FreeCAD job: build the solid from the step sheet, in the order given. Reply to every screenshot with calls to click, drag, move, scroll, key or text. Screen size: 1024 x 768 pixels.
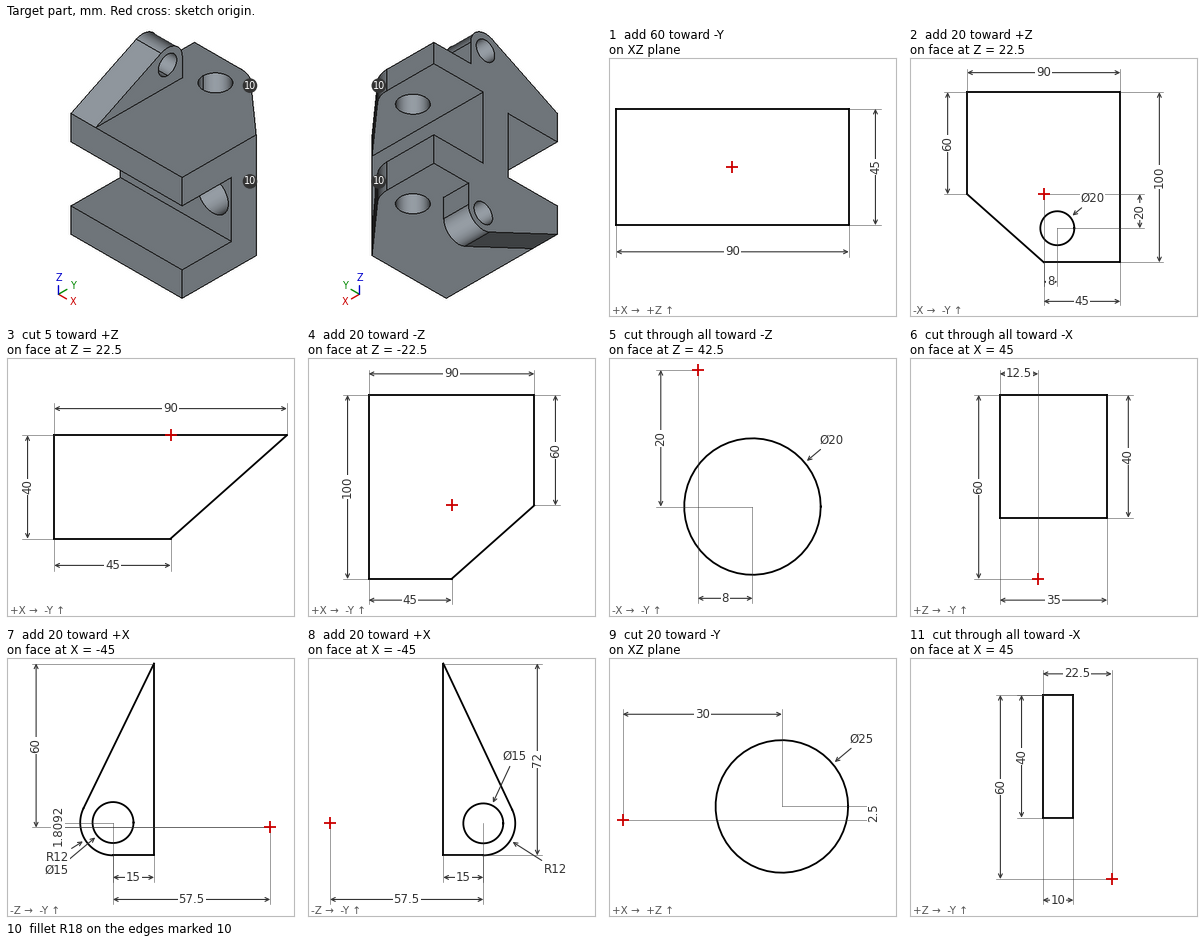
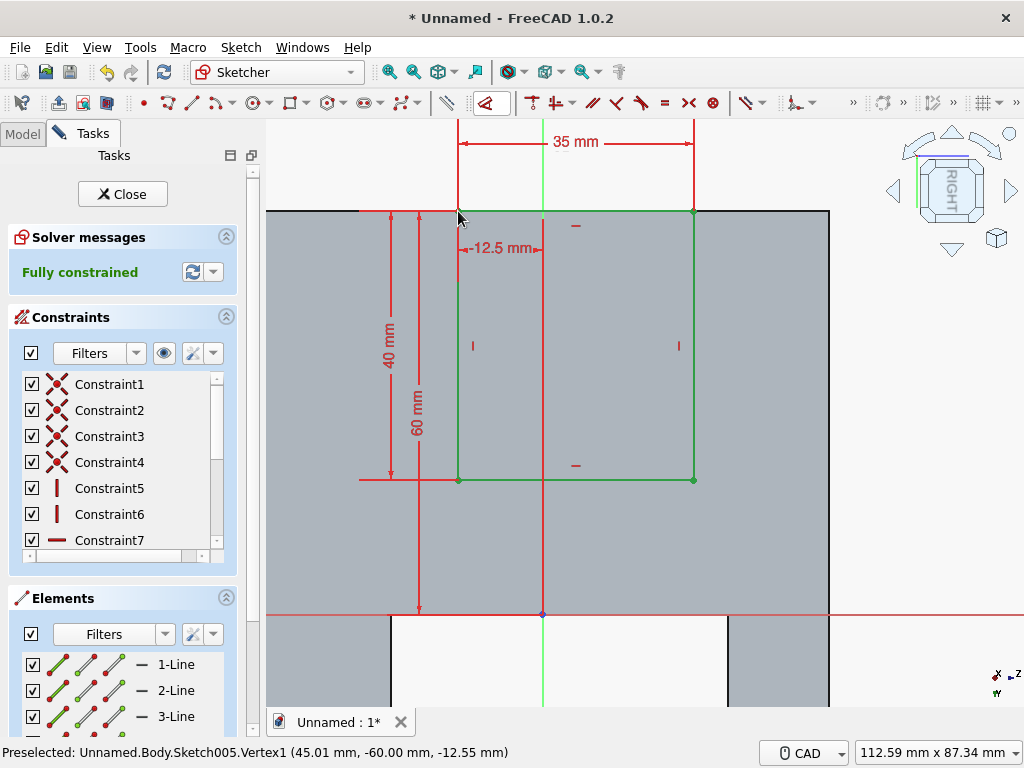
click(123, 194)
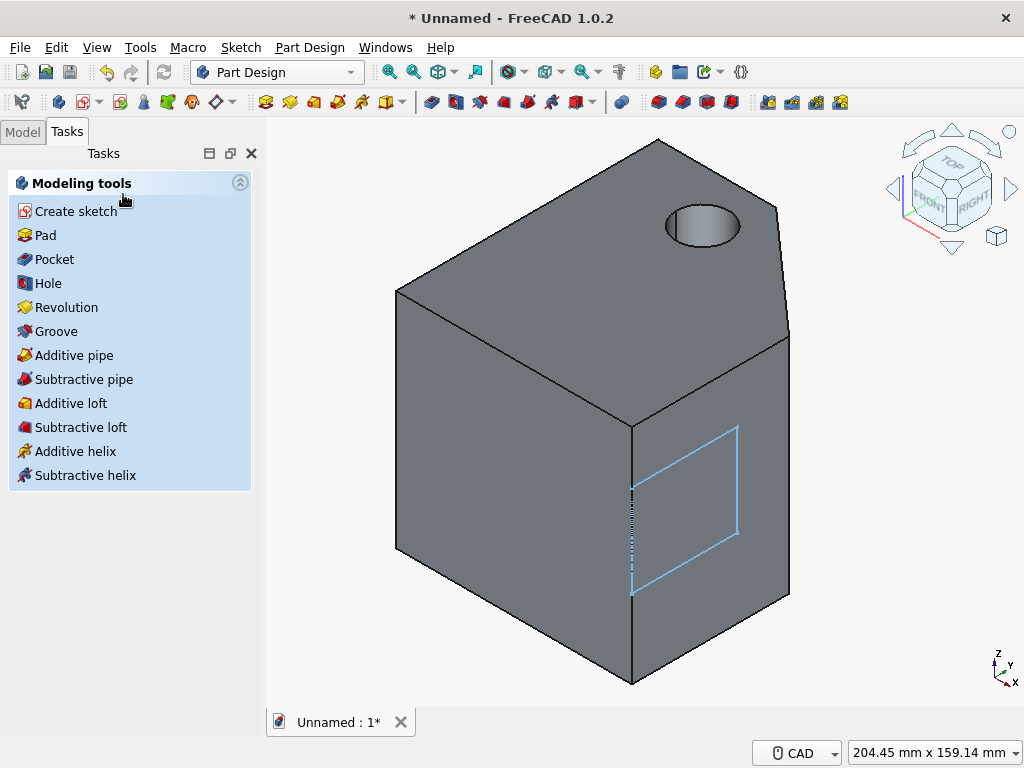
click(432, 102)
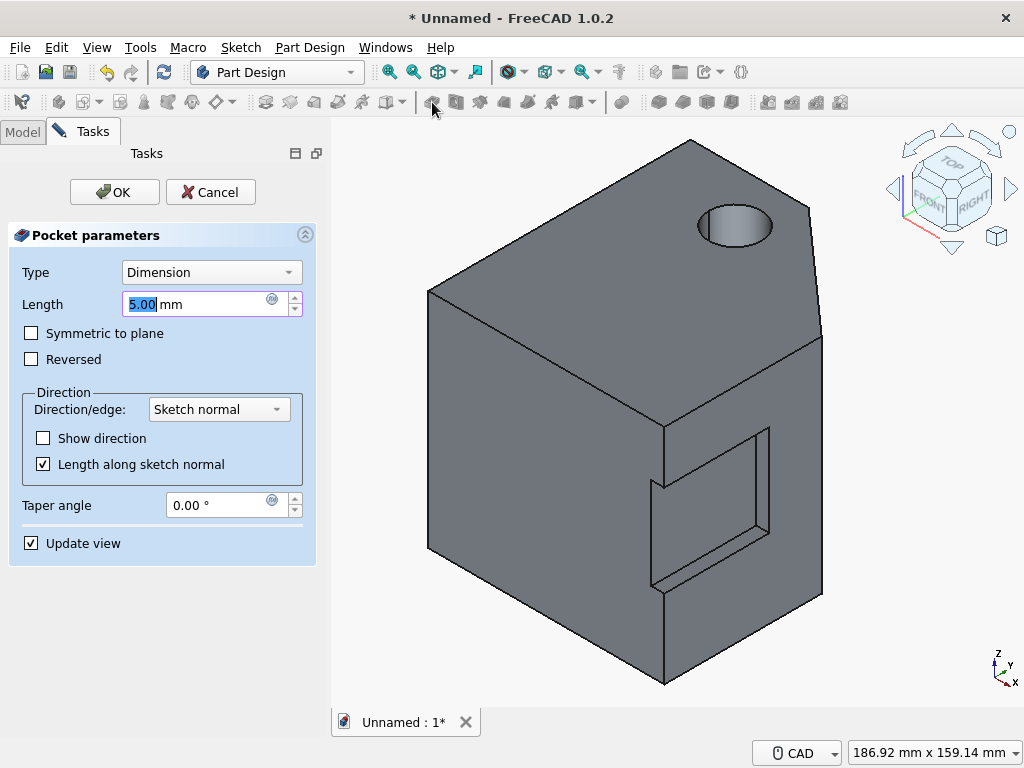
click(212, 272)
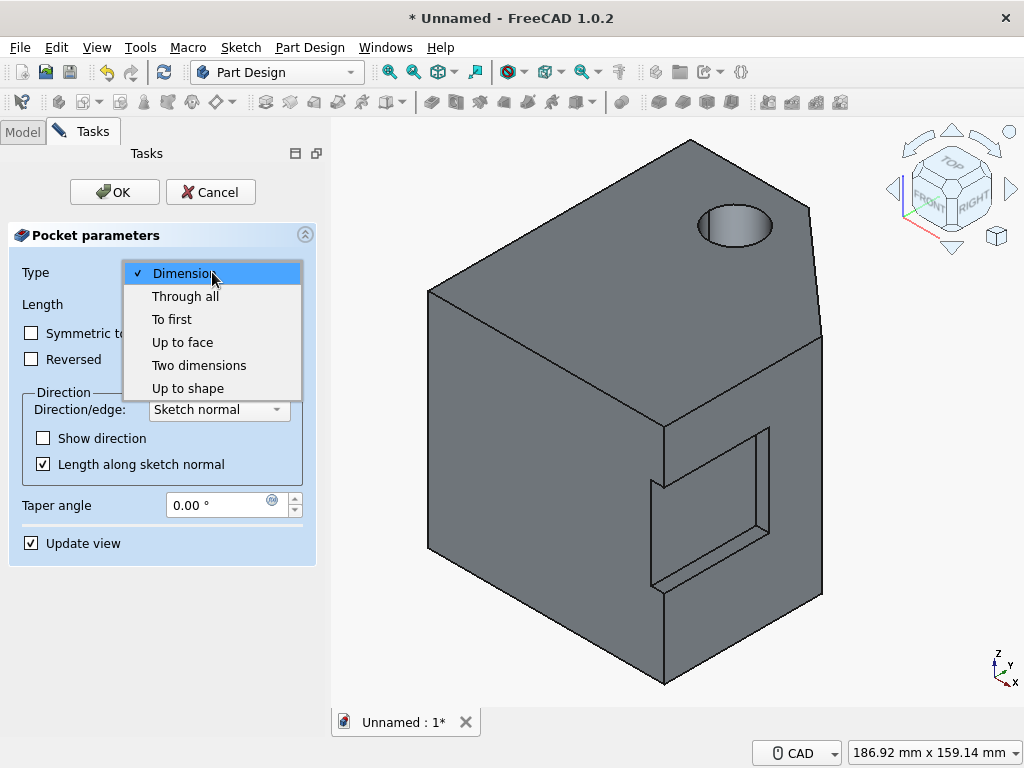
click(212, 296)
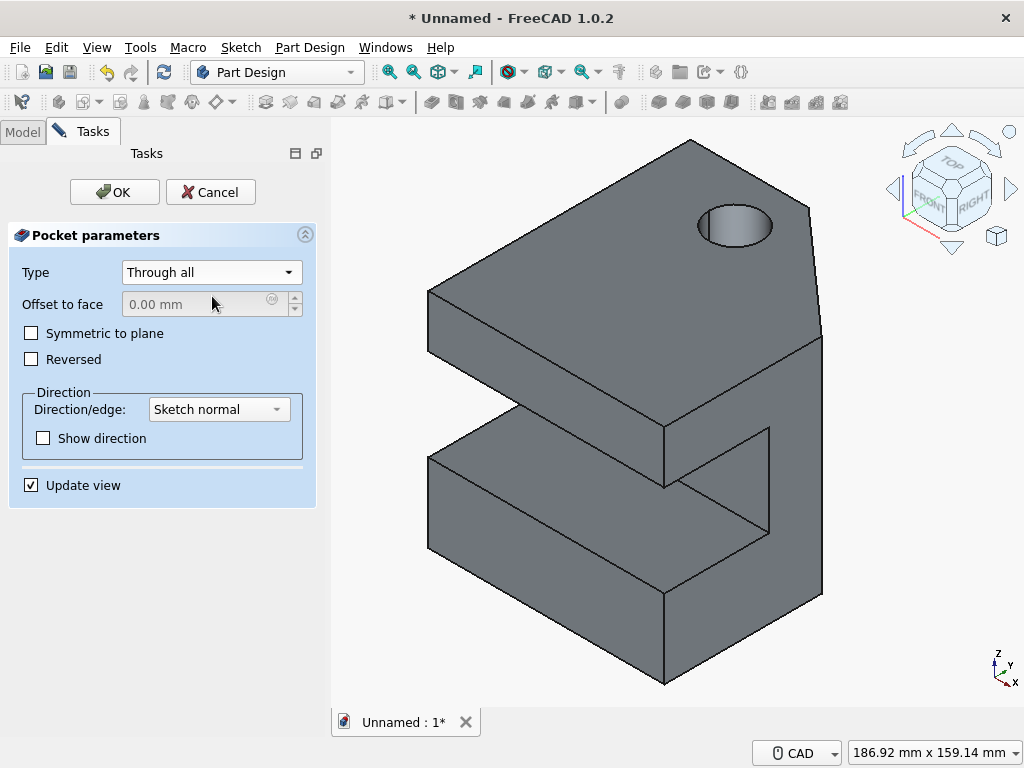
click(115, 192)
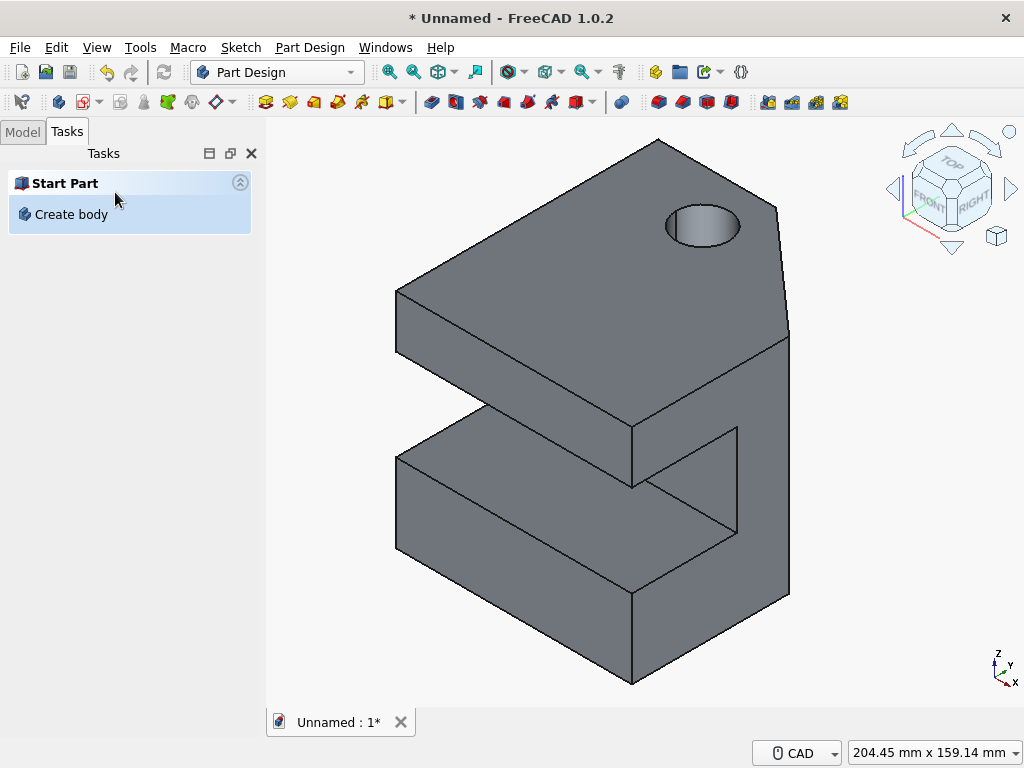
key(6)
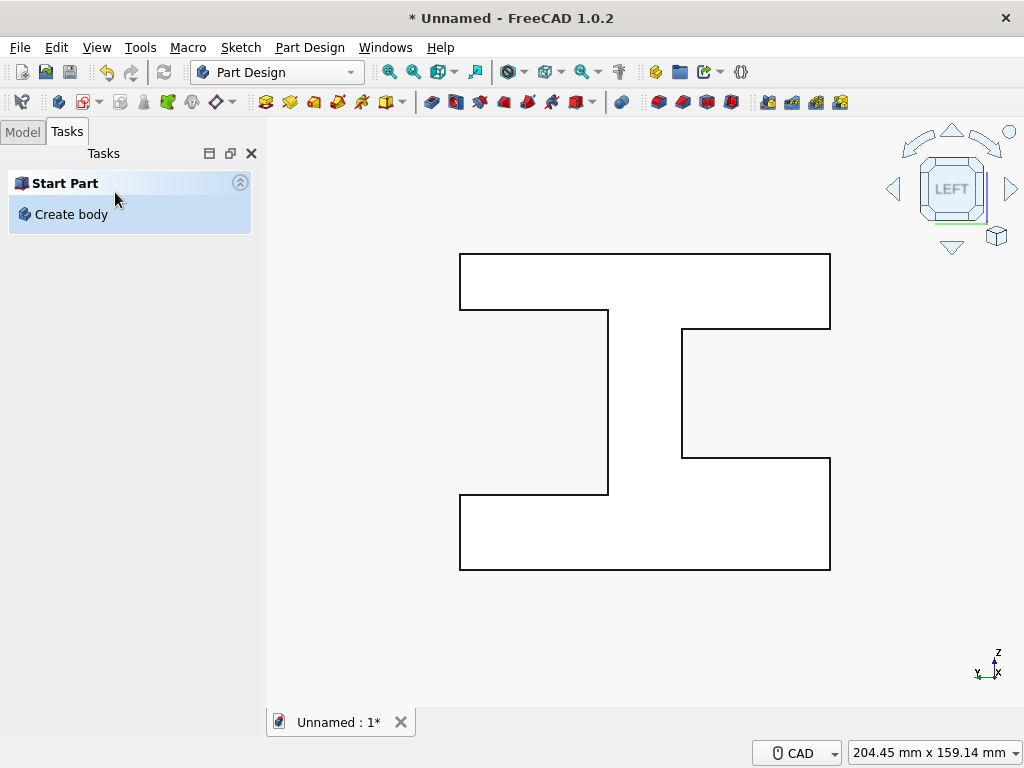
click(698, 501)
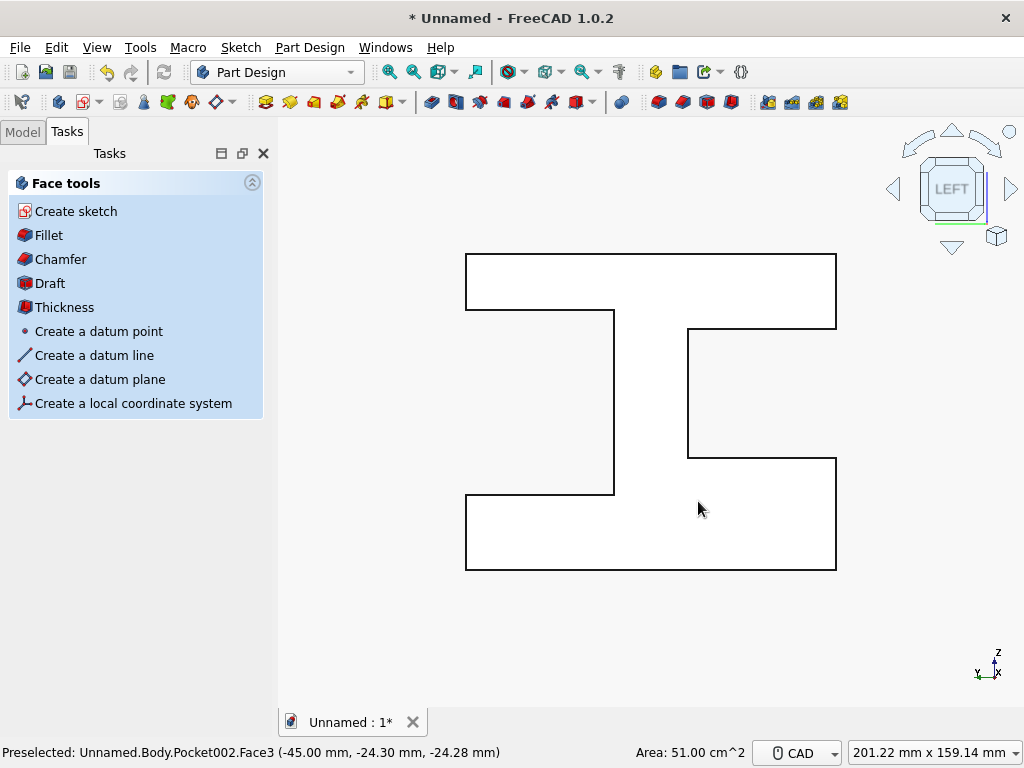
click(84, 102)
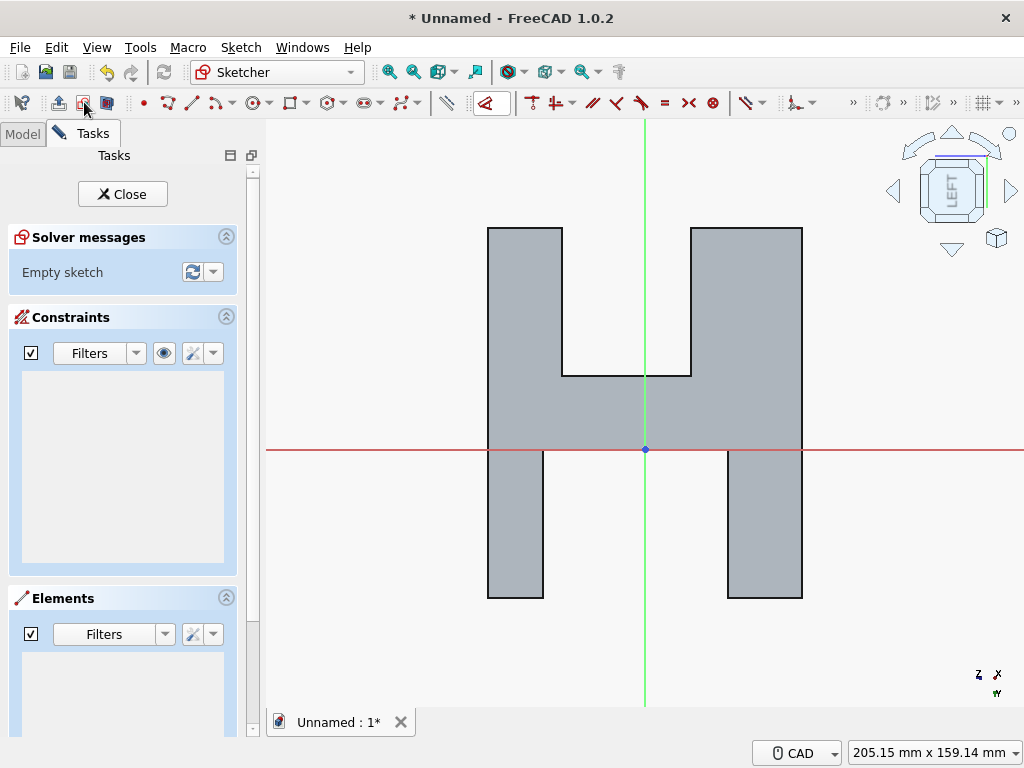
scroll(402, 246, up, 2)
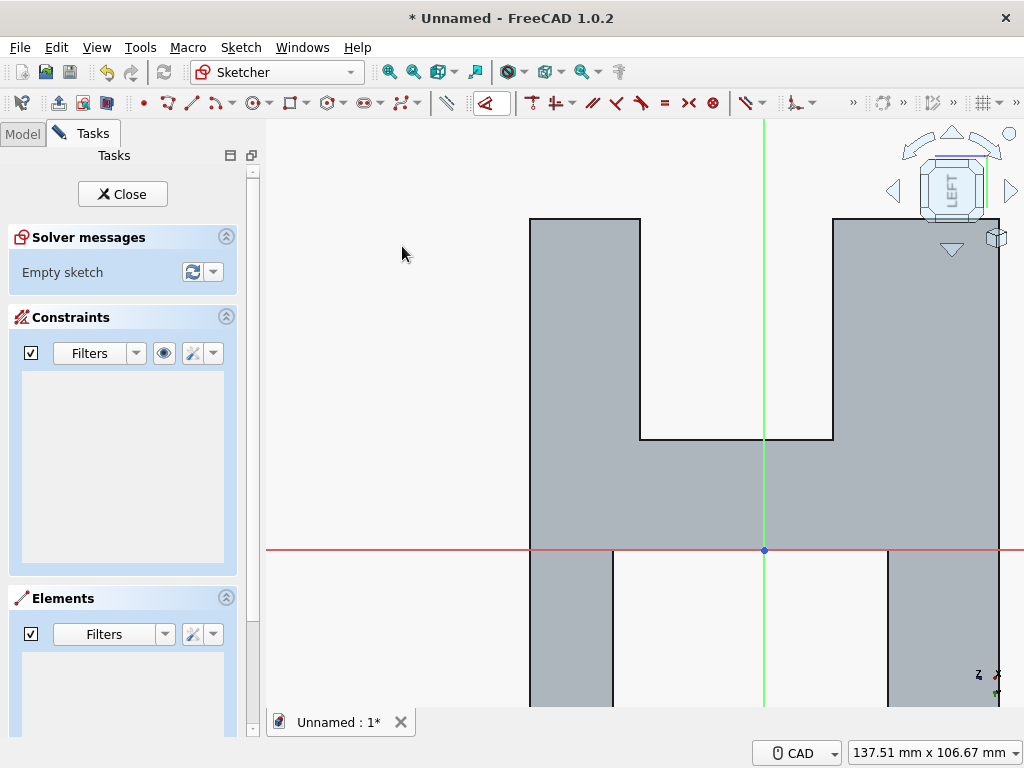
key(g)
key(m)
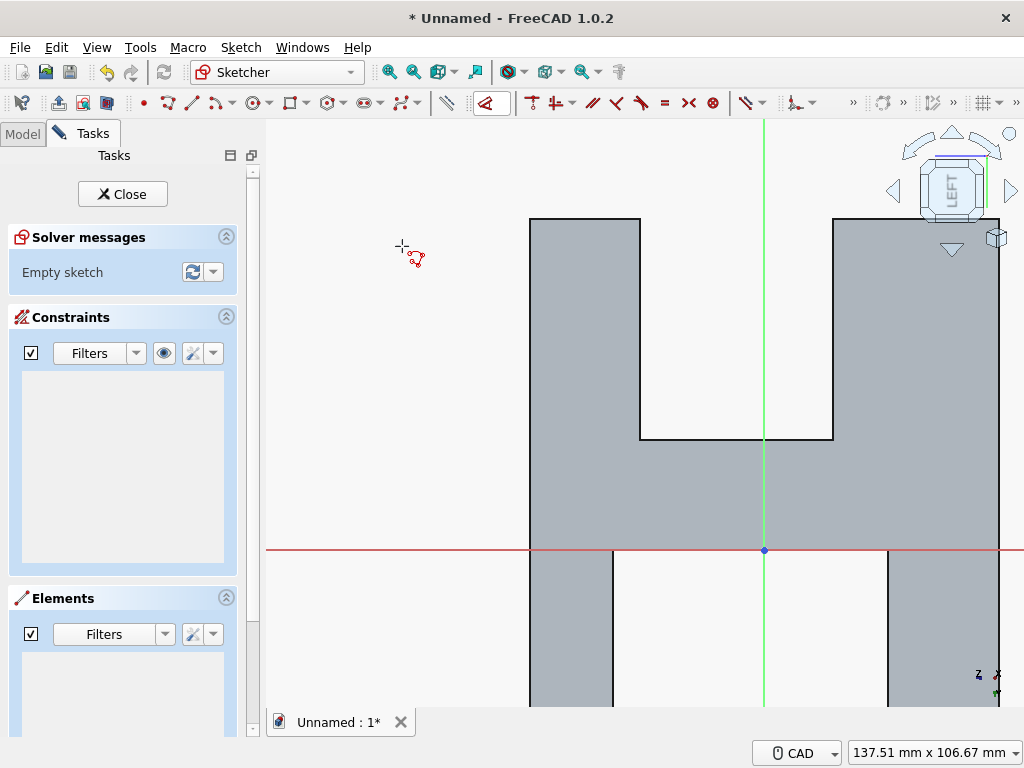
click(447, 606)
click(530, 606)
click(530, 219)
click(388, 511)
right_click(388, 511)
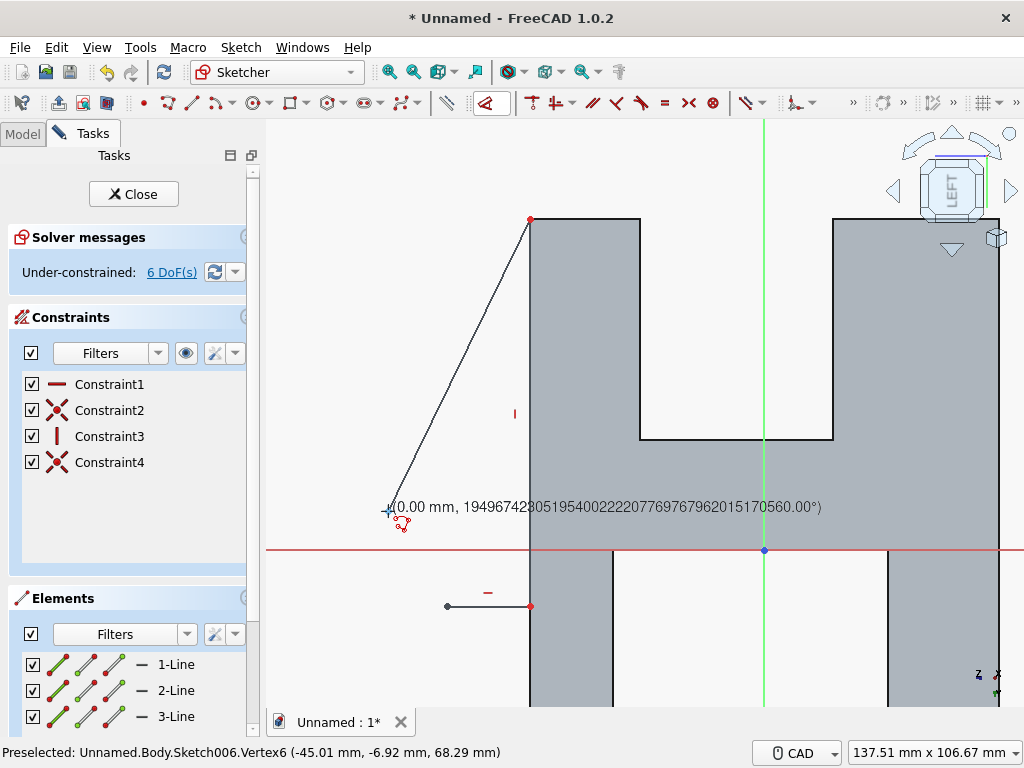
key(g)
key(3)
key(a)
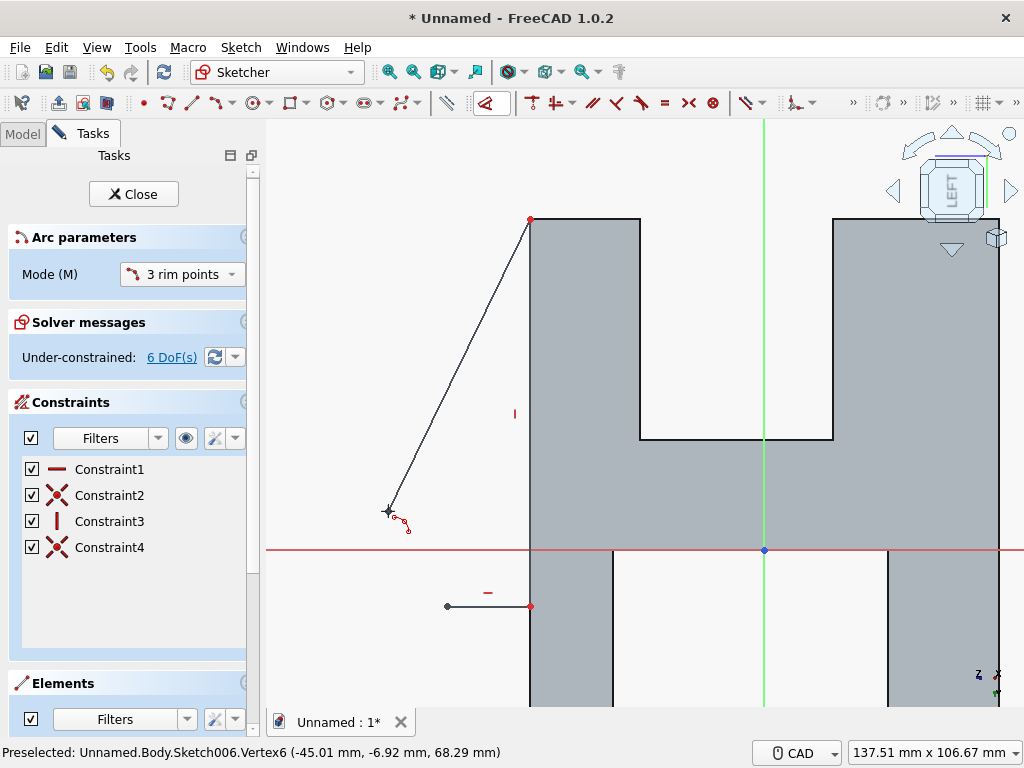
click(388, 512)
click(447, 607)
click(391, 575)